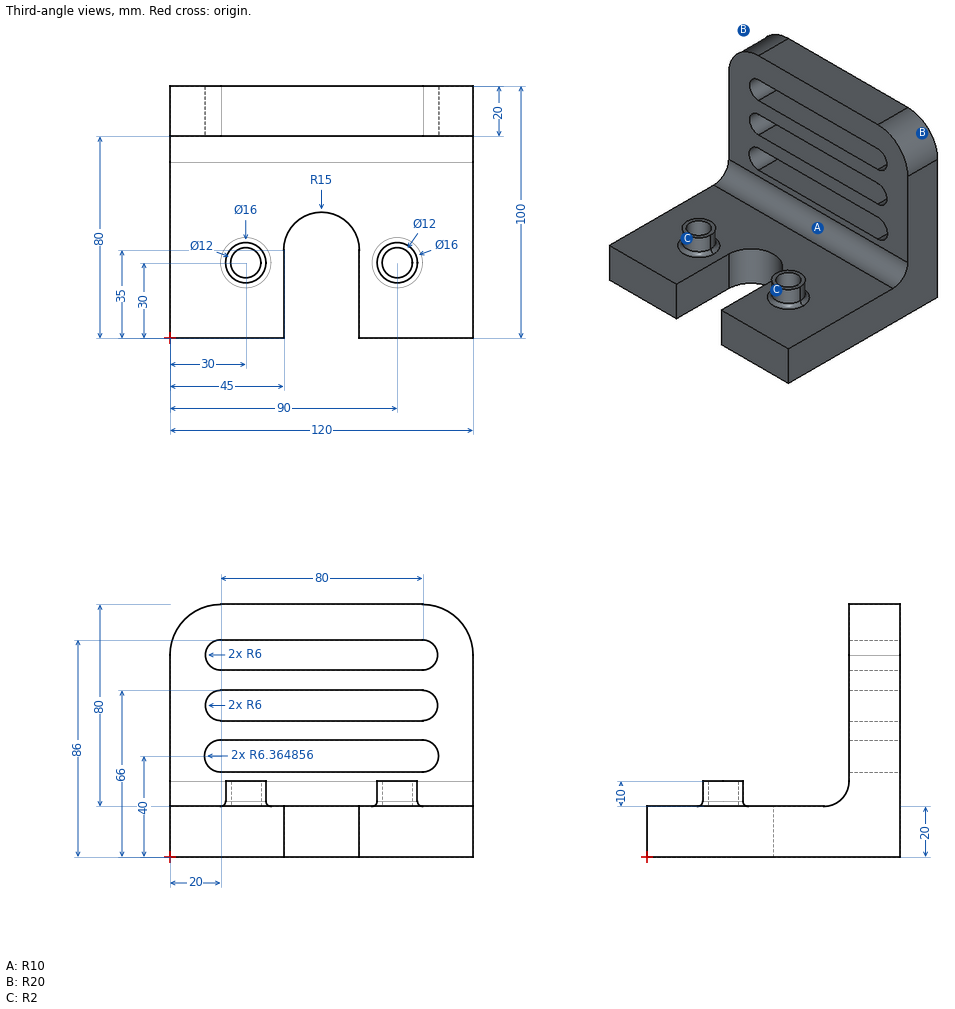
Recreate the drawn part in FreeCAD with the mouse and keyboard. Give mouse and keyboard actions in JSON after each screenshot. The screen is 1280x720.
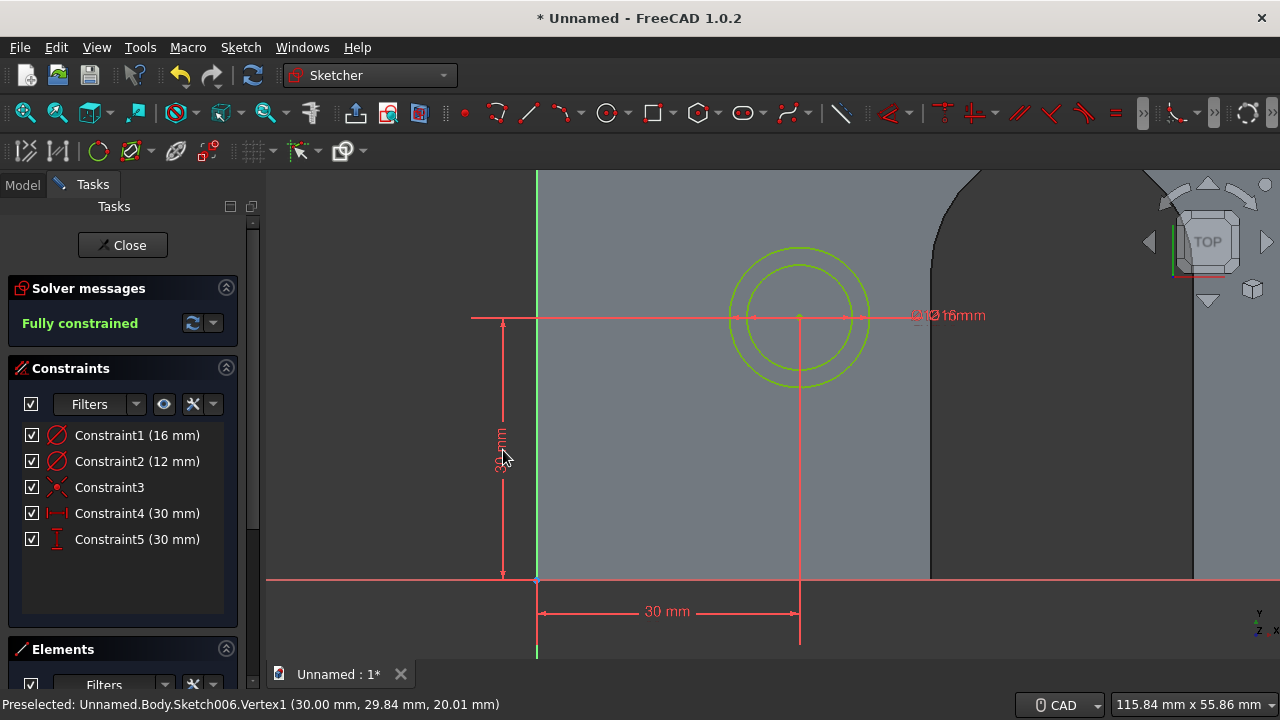
{"action": "left_click", "coordinate": [123, 245]}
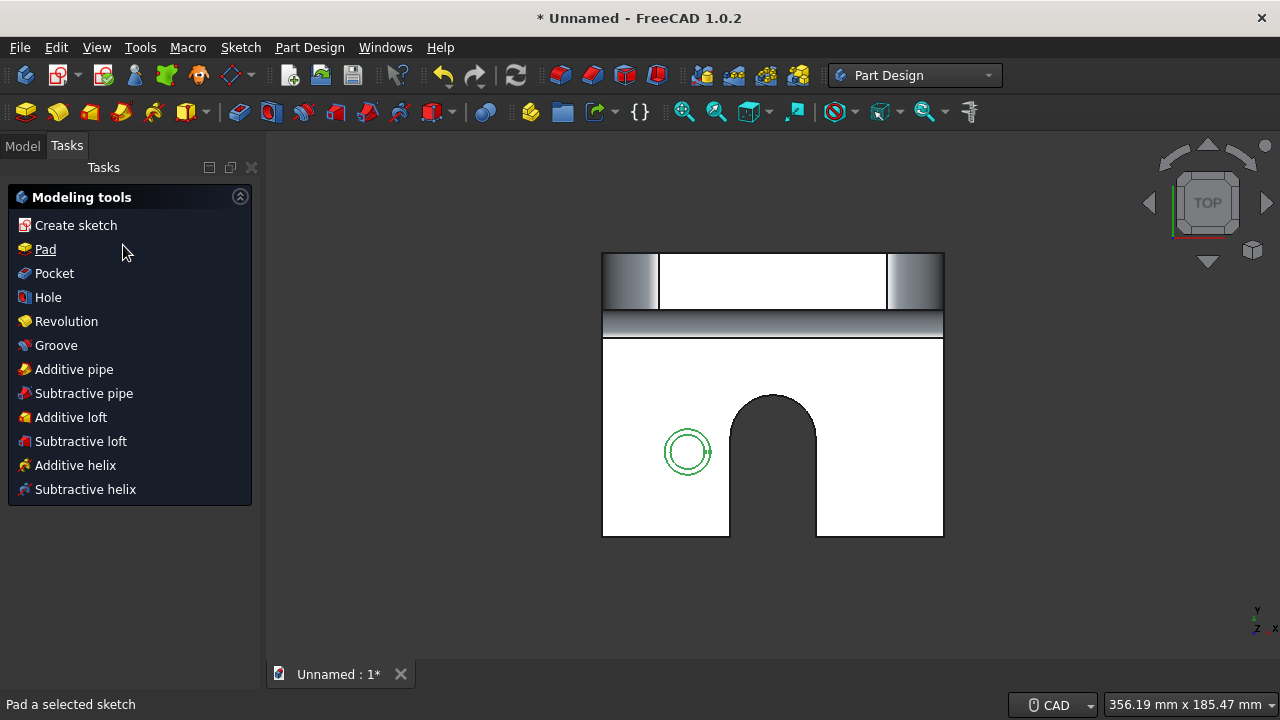
{"action": "left_click", "coordinate": [26, 112]}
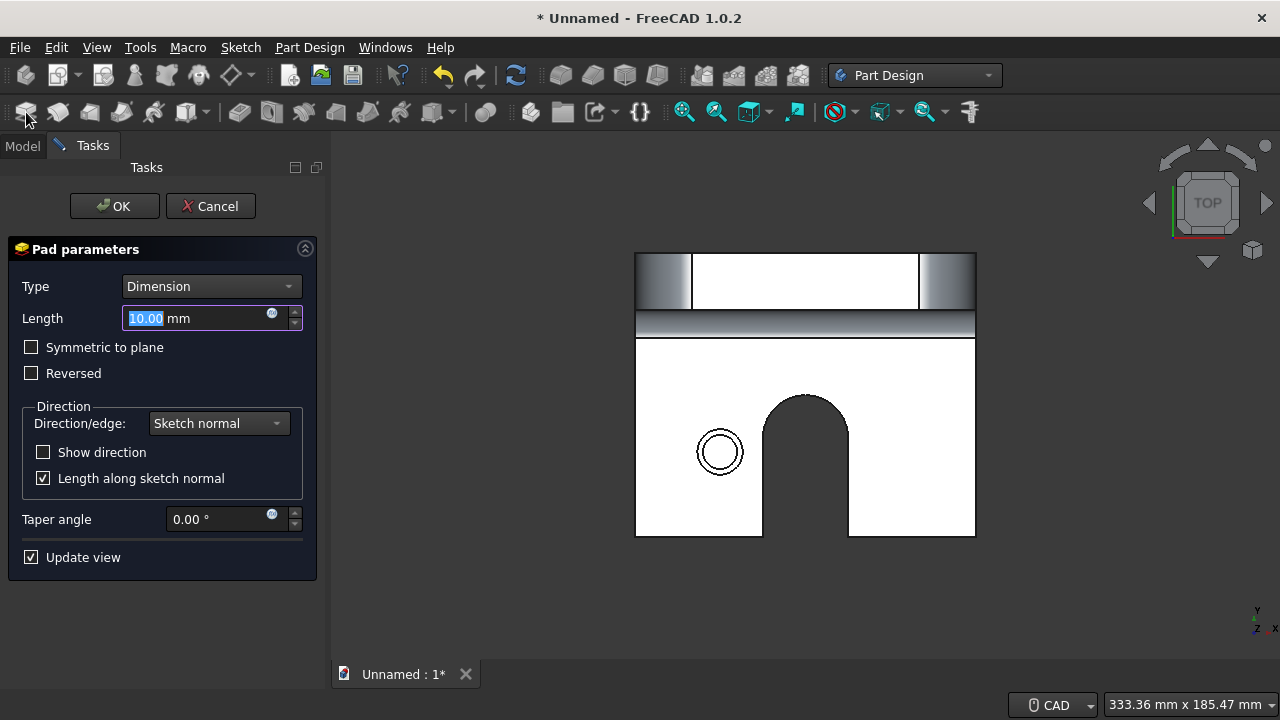
{"action": "type", "text": "10"}
{"action": "key", "text": "Tab"}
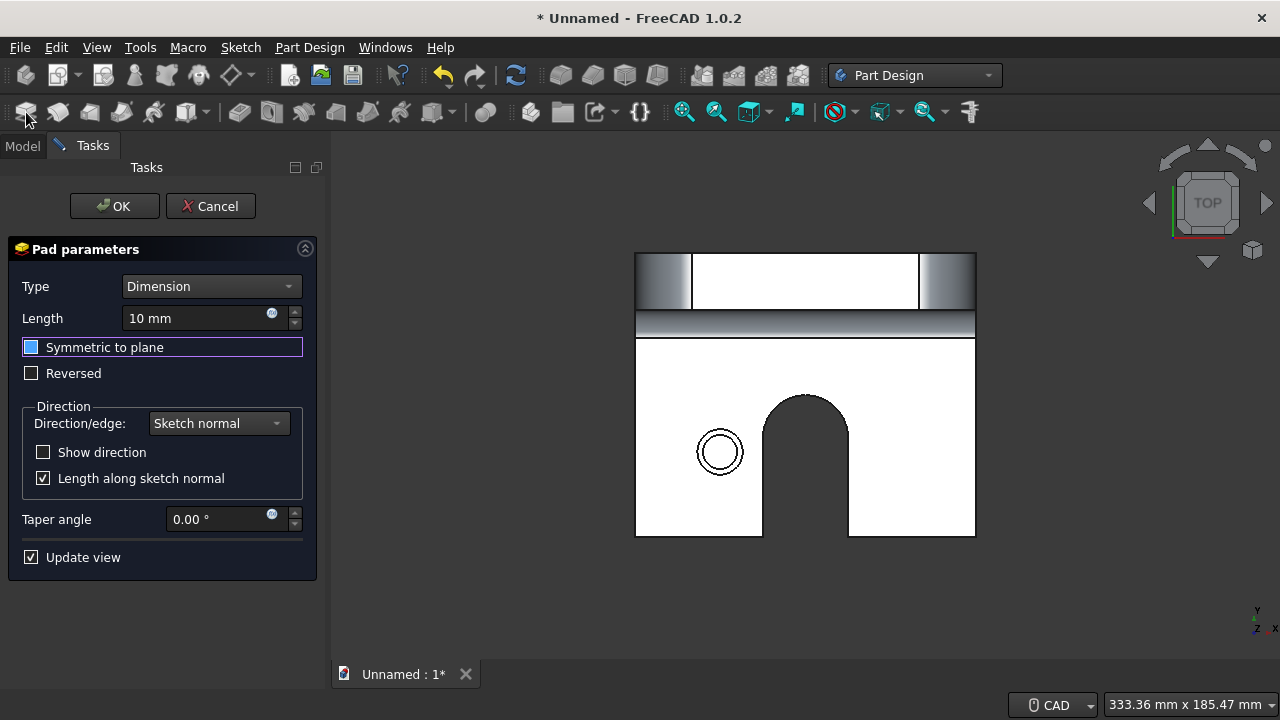
{"action": "left_click", "coordinate": [115, 206]}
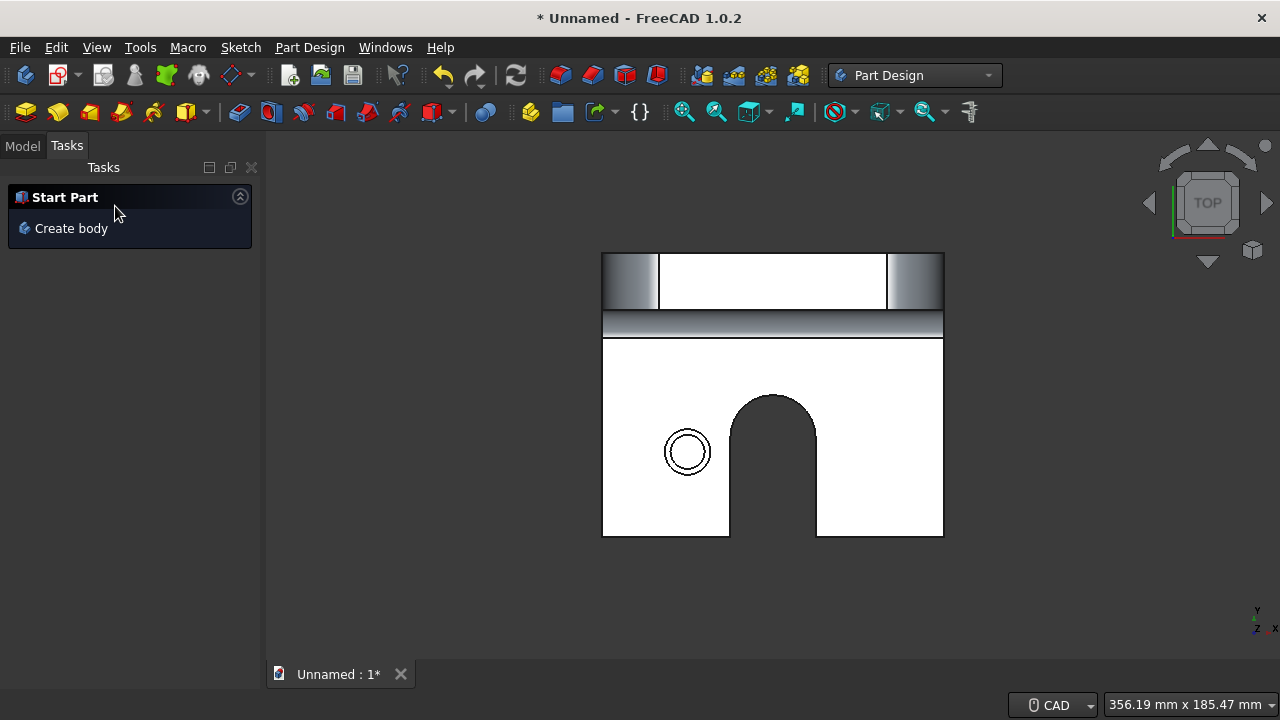
{"action": "left_click", "coordinate": [871, 408]}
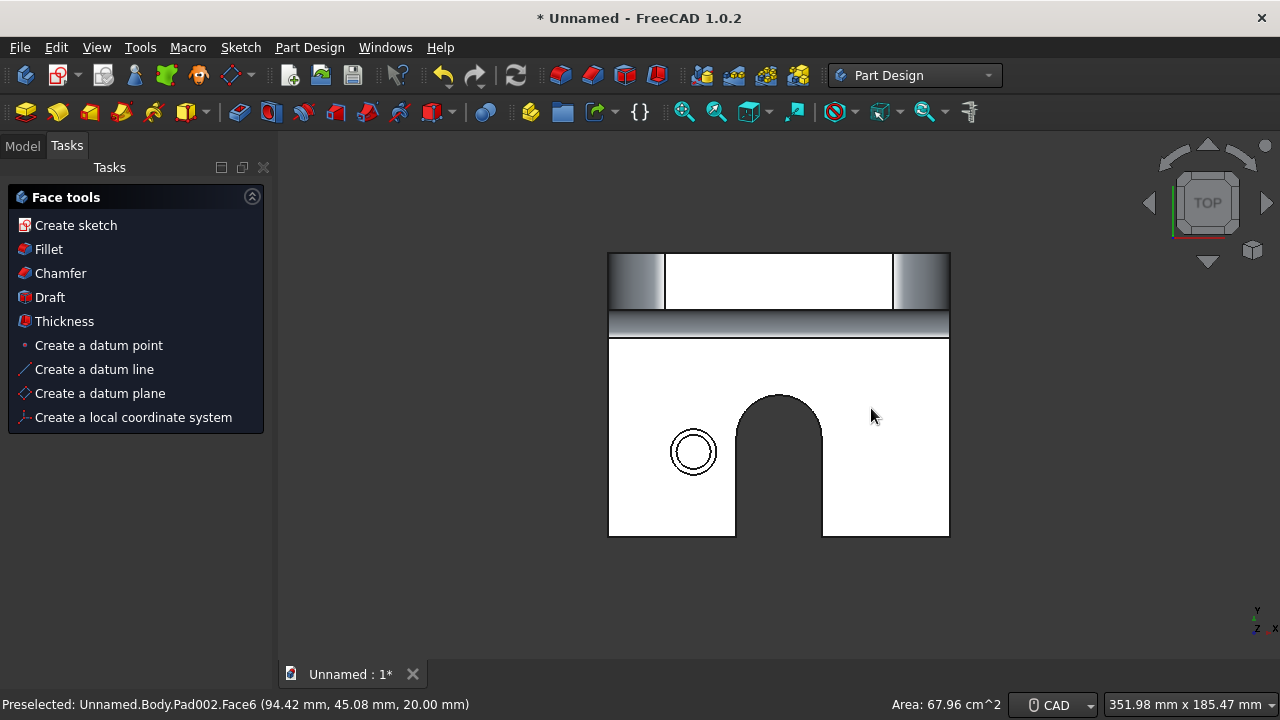
{"action": "left_click", "coordinate": [58, 76]}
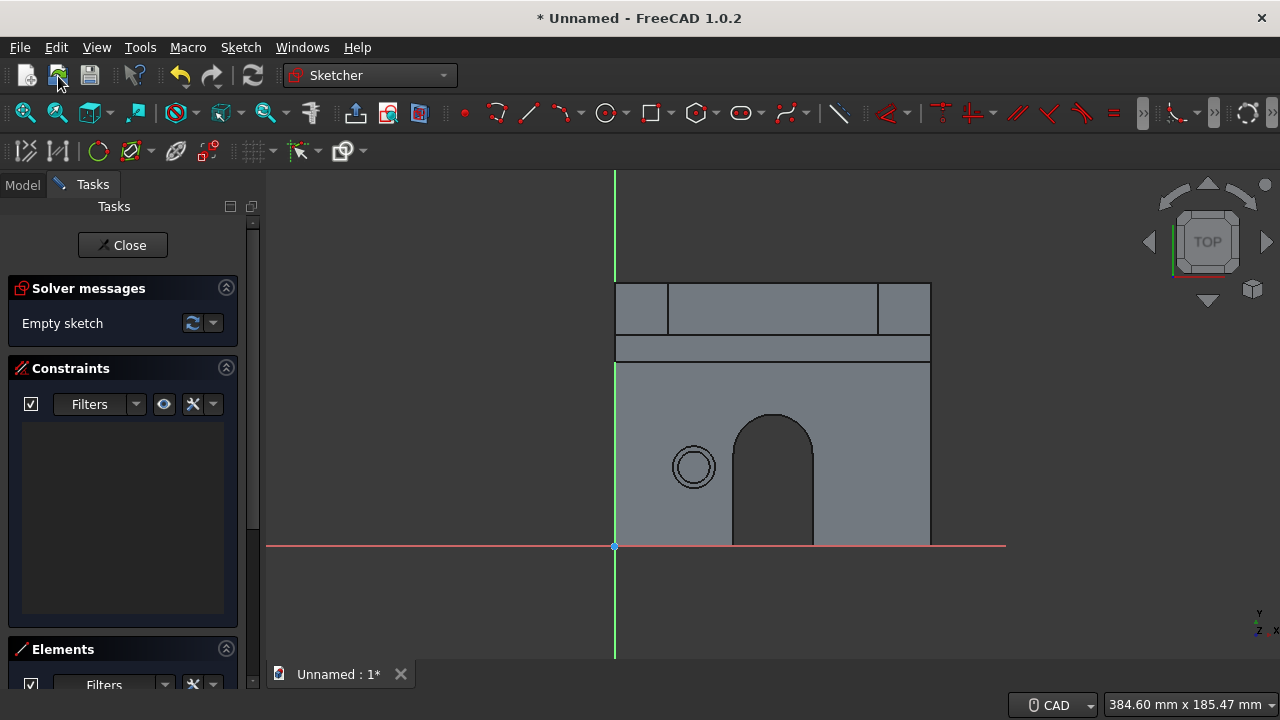
{"action": "scroll", "coordinate": [875, 475], "scroll_direction": "up", "scroll_amount": 10}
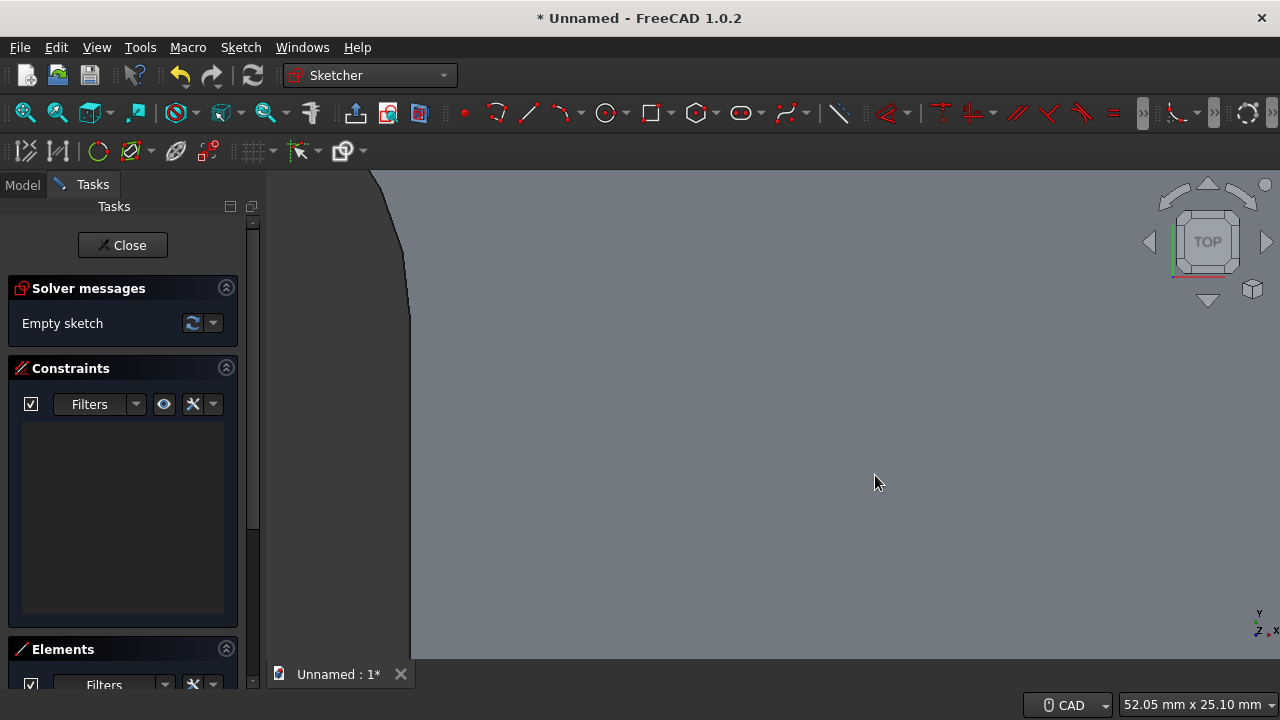
{"action": "key", "text": "g c"}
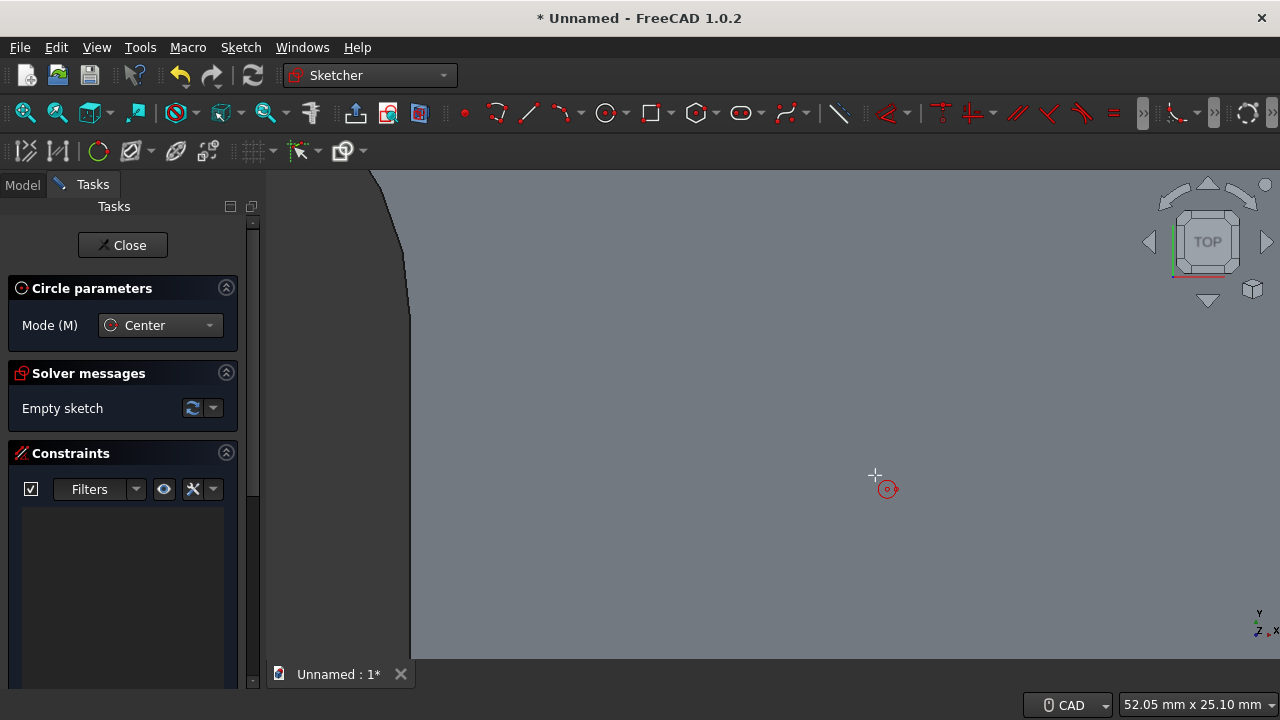
{"action": "left_click", "coordinate": [702, 414]}
{"action": "mouse_move", "coordinate": [812, 303]}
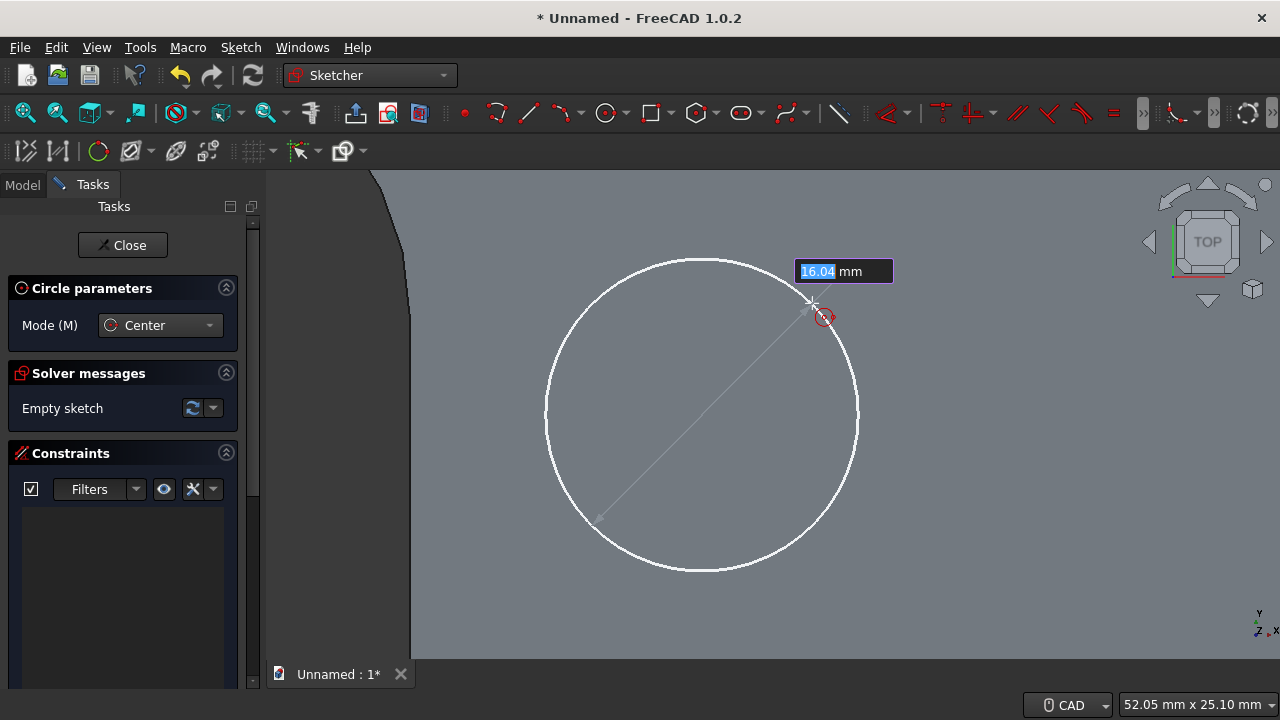
{"action": "type", "text": "16"}
{"action": "key", "text": "Return"}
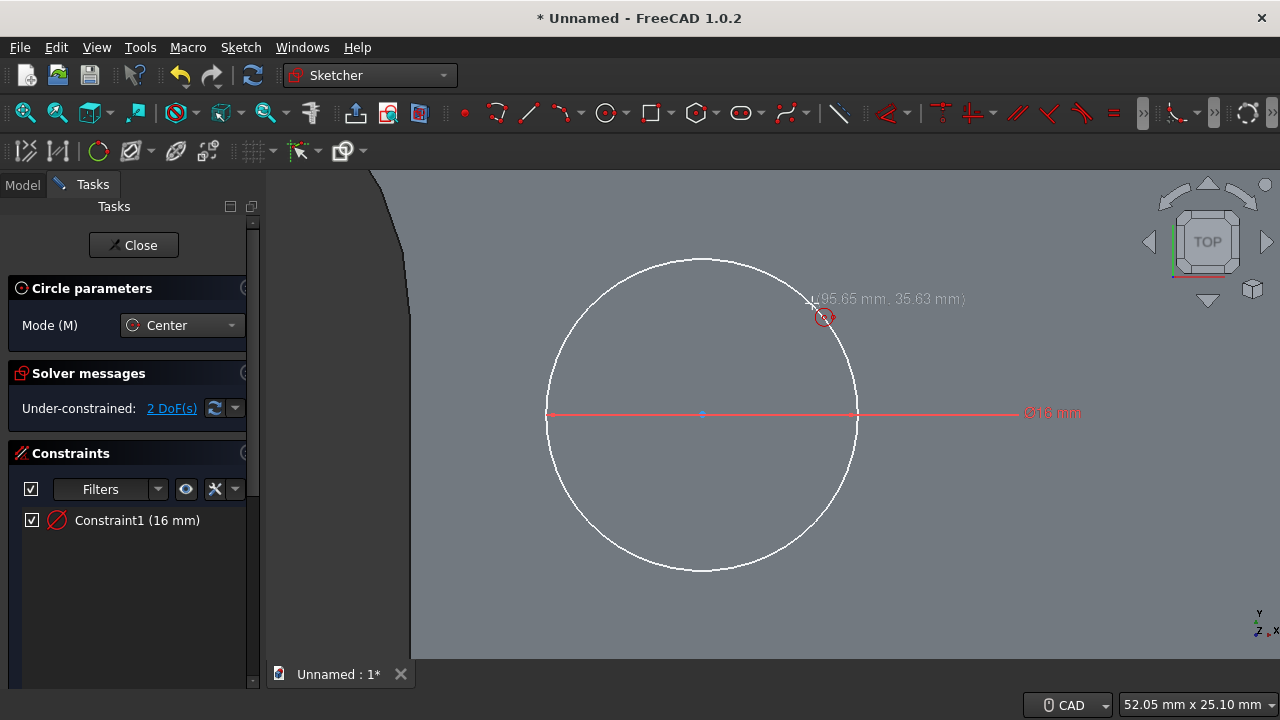
{"action": "left_click", "coordinate": [702, 415]}
{"action": "mouse_move", "coordinate": [785, 331]}